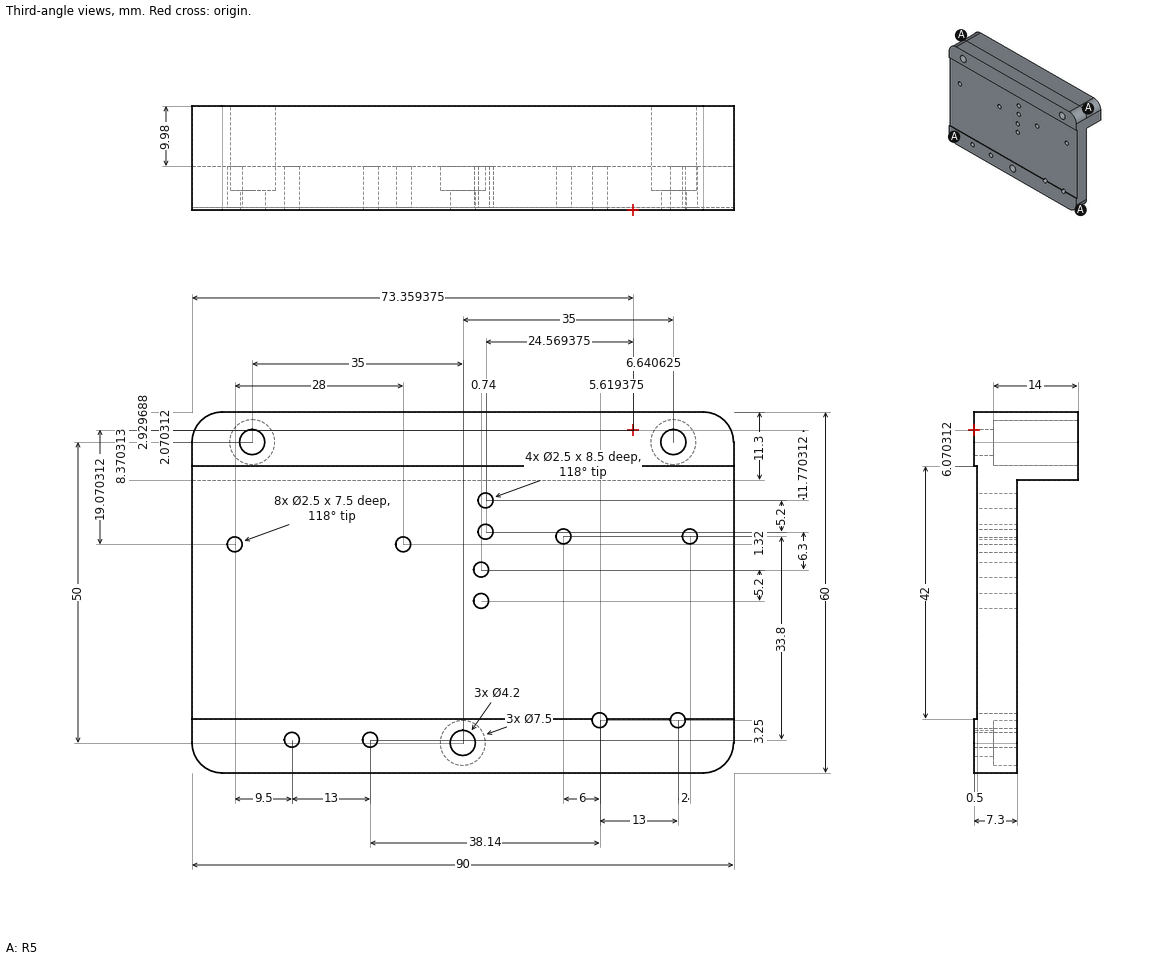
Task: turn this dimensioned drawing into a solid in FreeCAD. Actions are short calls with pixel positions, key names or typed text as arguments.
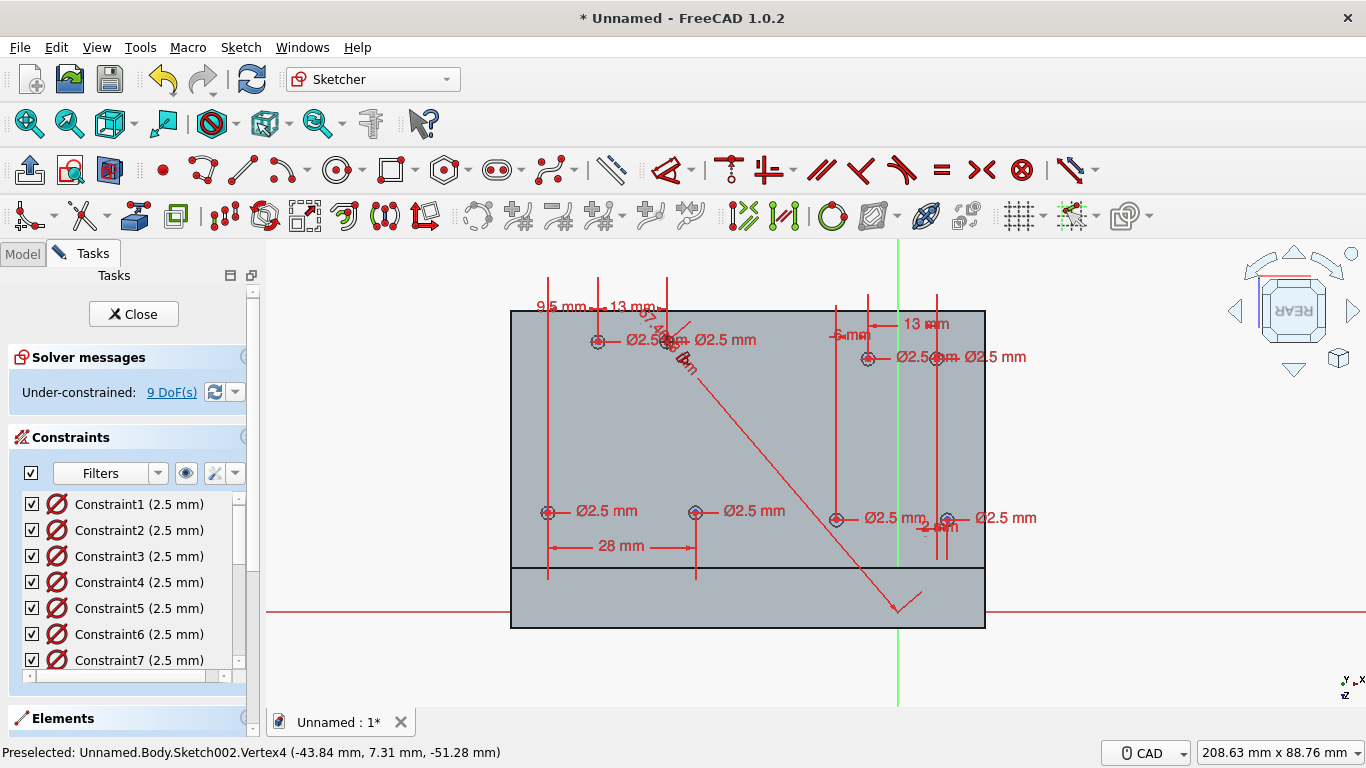
scroll(868, 359, up, 5)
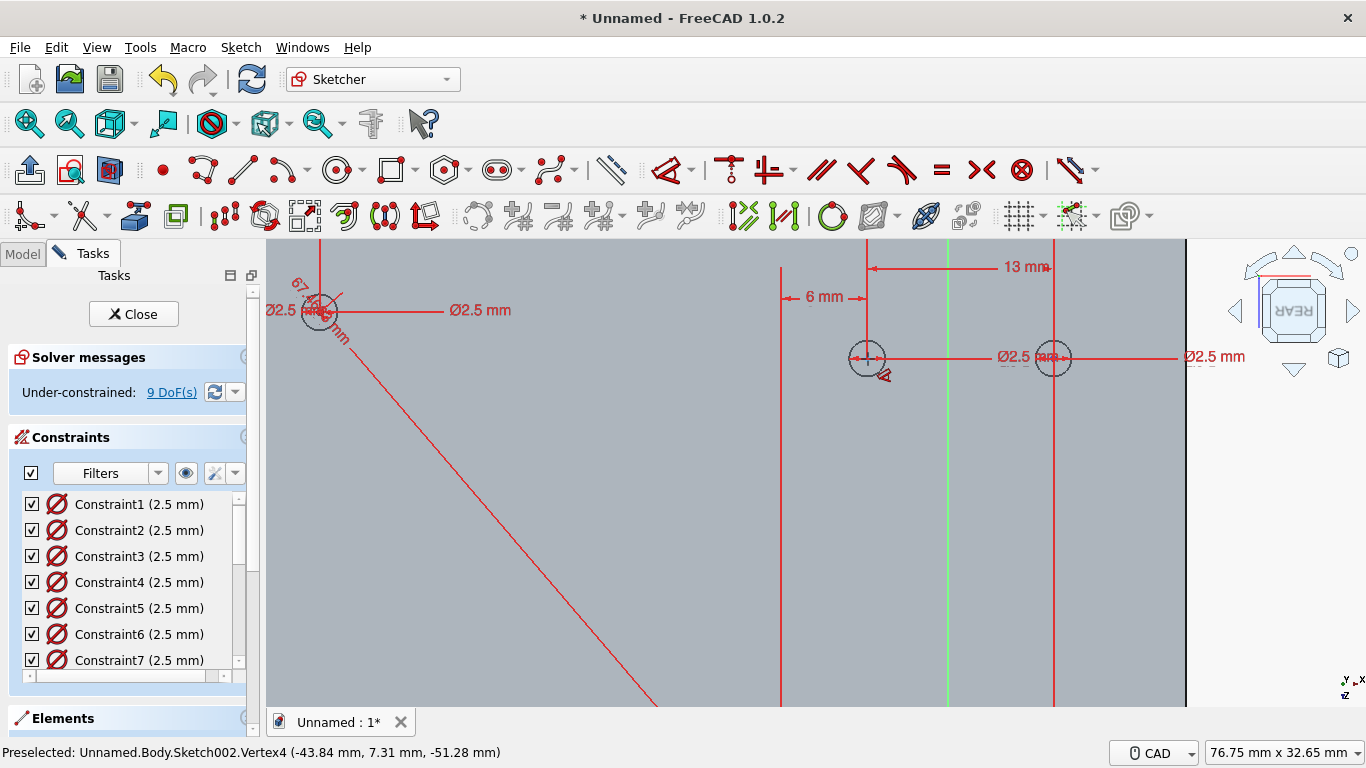
click(867, 359)
click(901, 335)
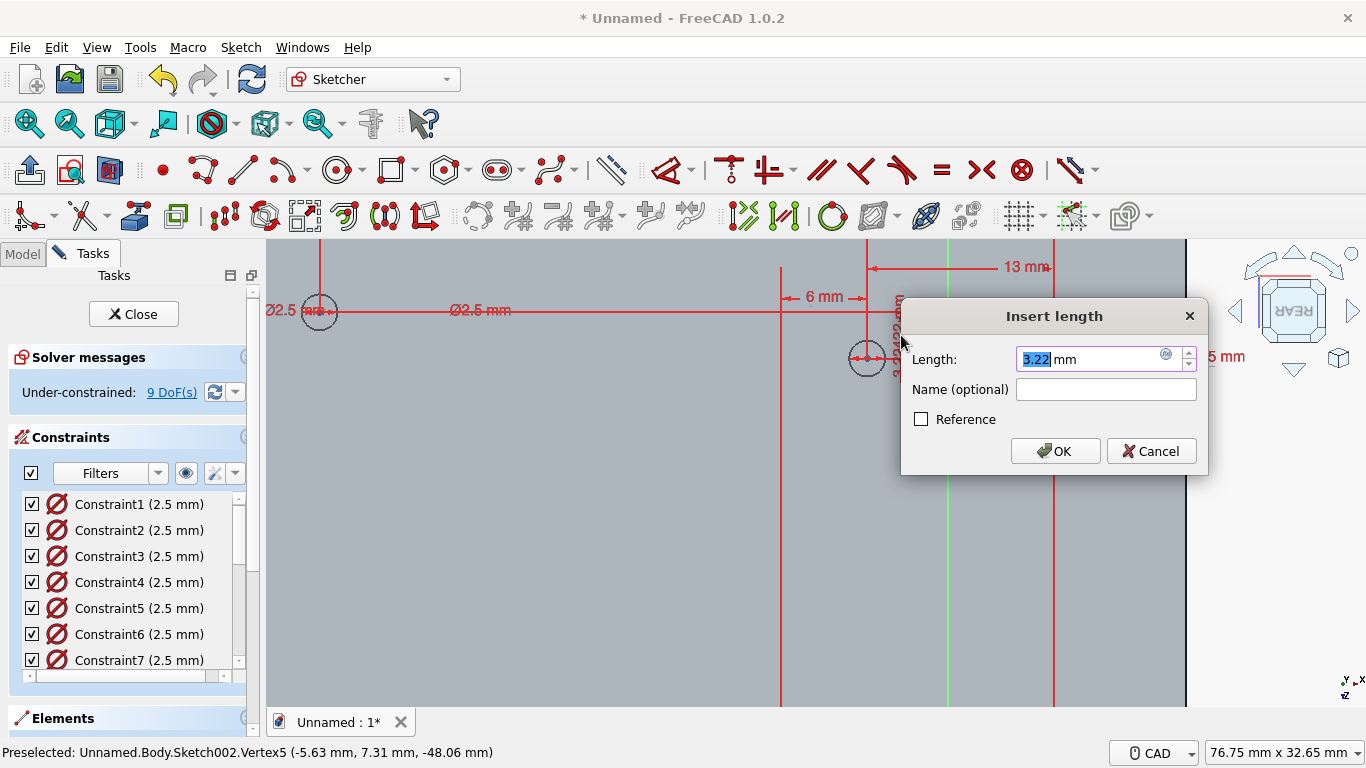
text(3.25)
key(Return)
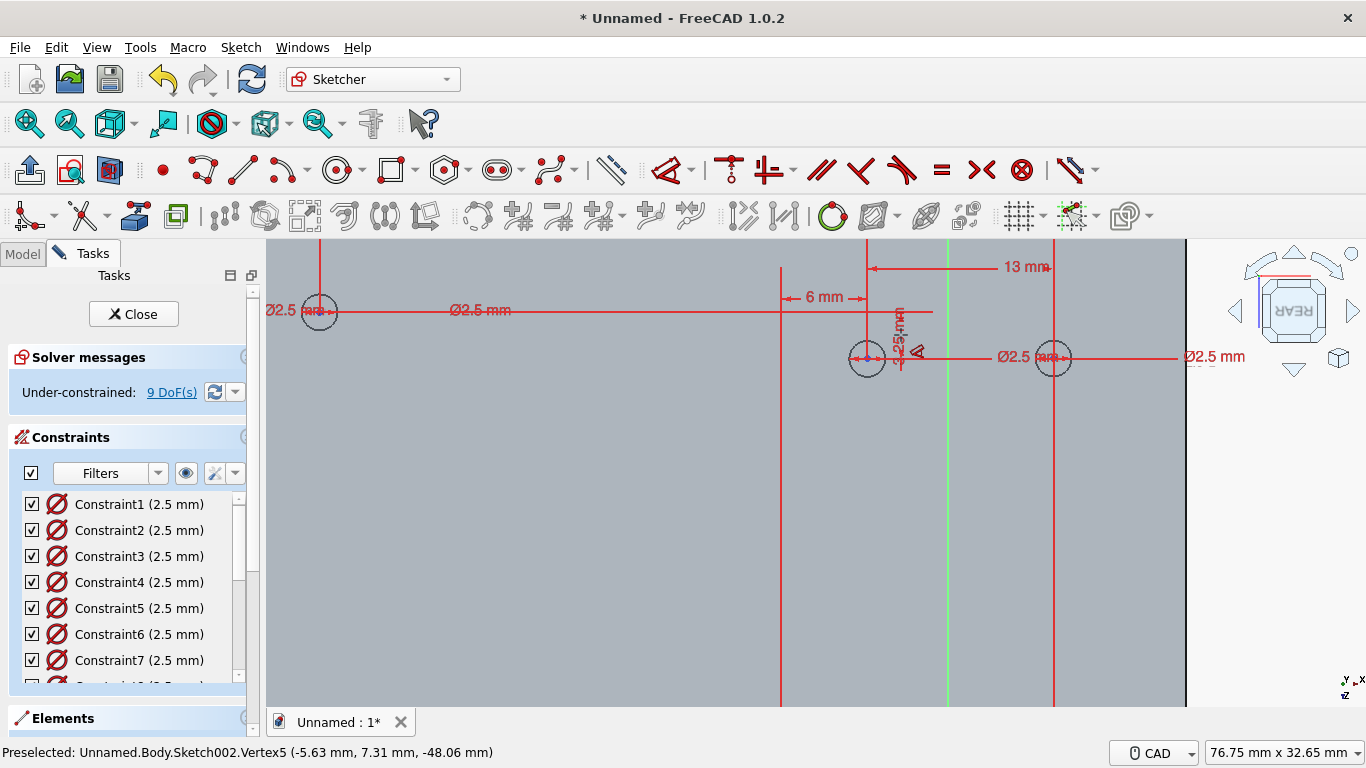
scroll(868, 359, down, 5)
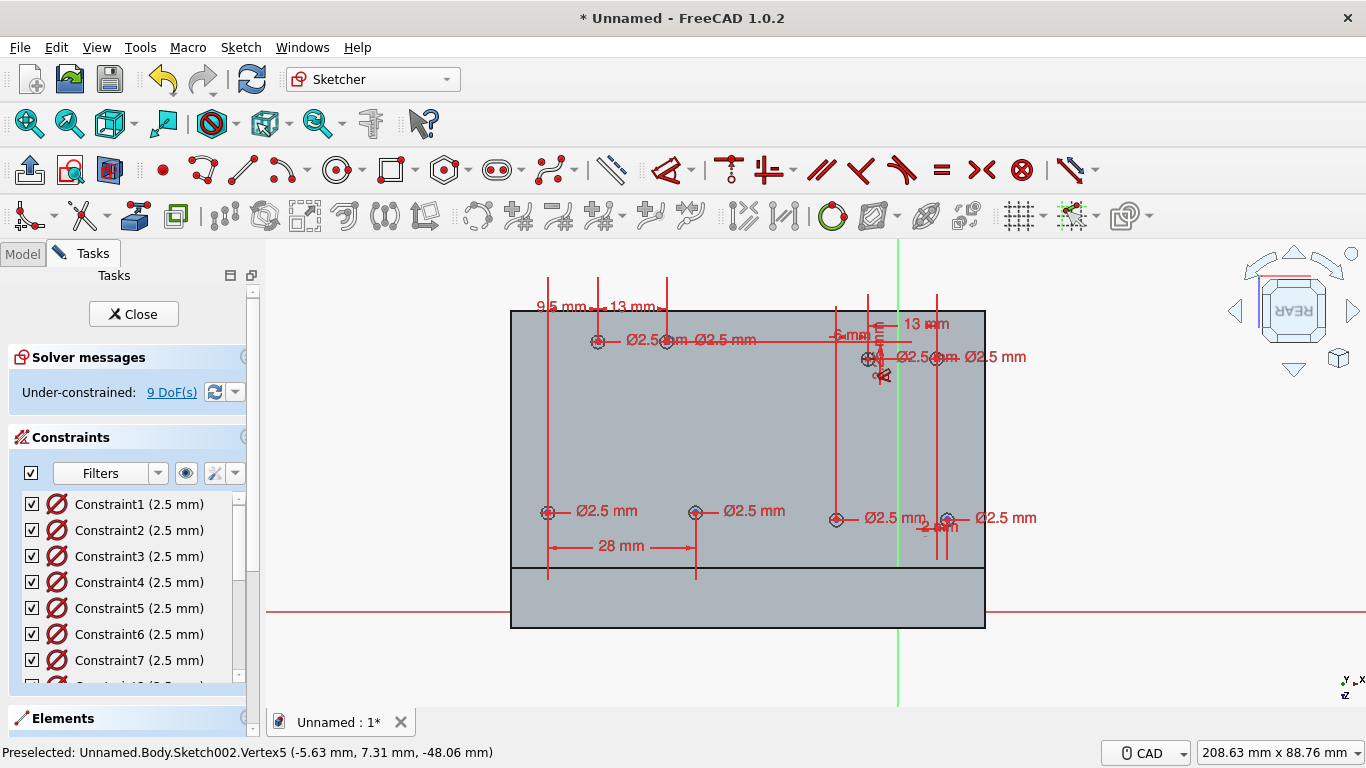
scroll(598, 342, up, 5)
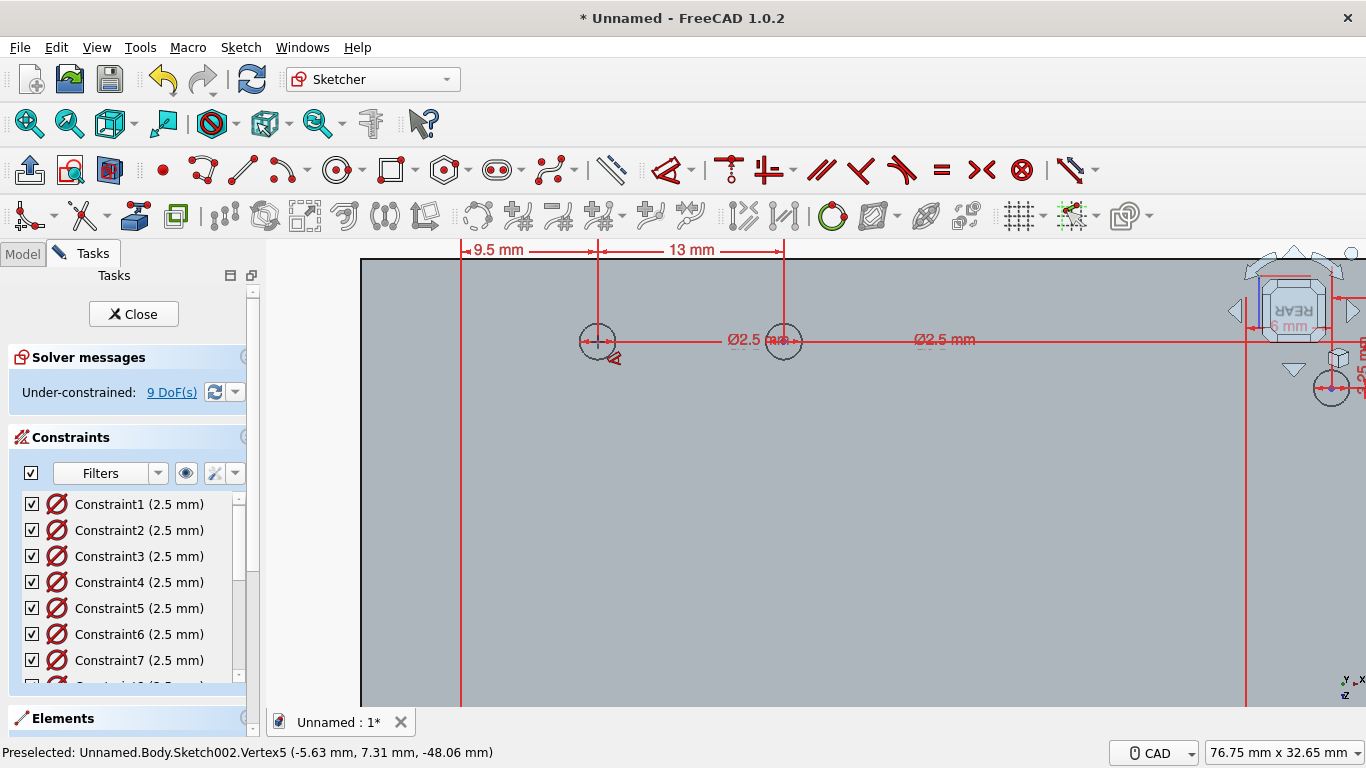
click(598, 342)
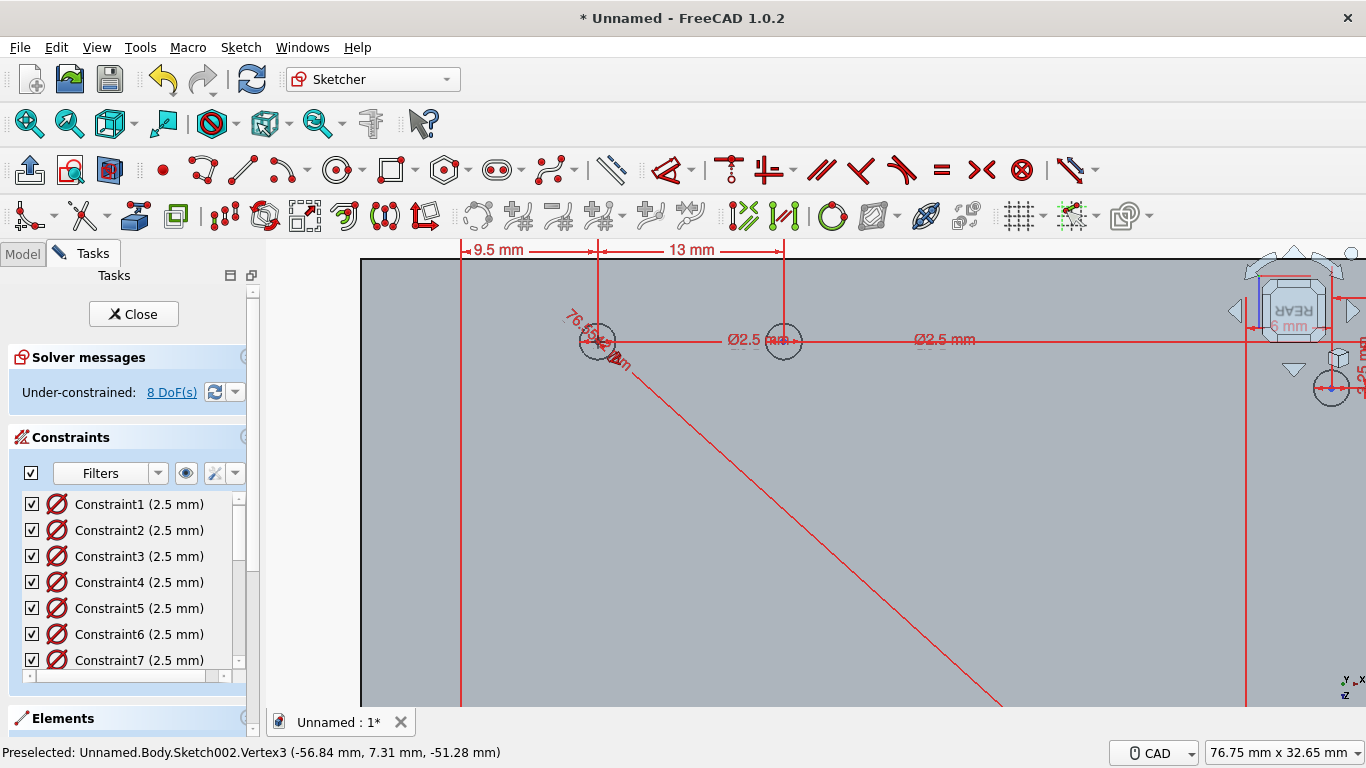
scroll(598, 342, down, 5)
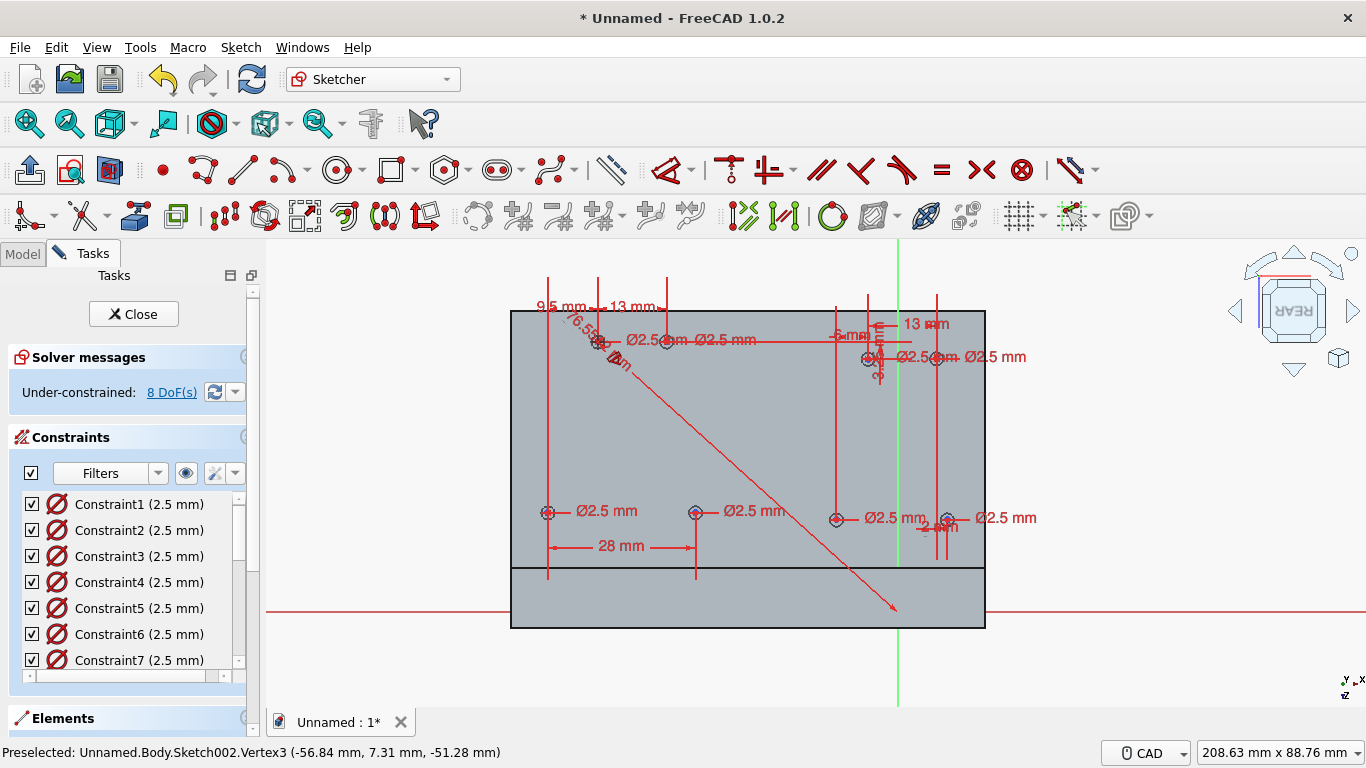
scroll(868, 359, up, 5)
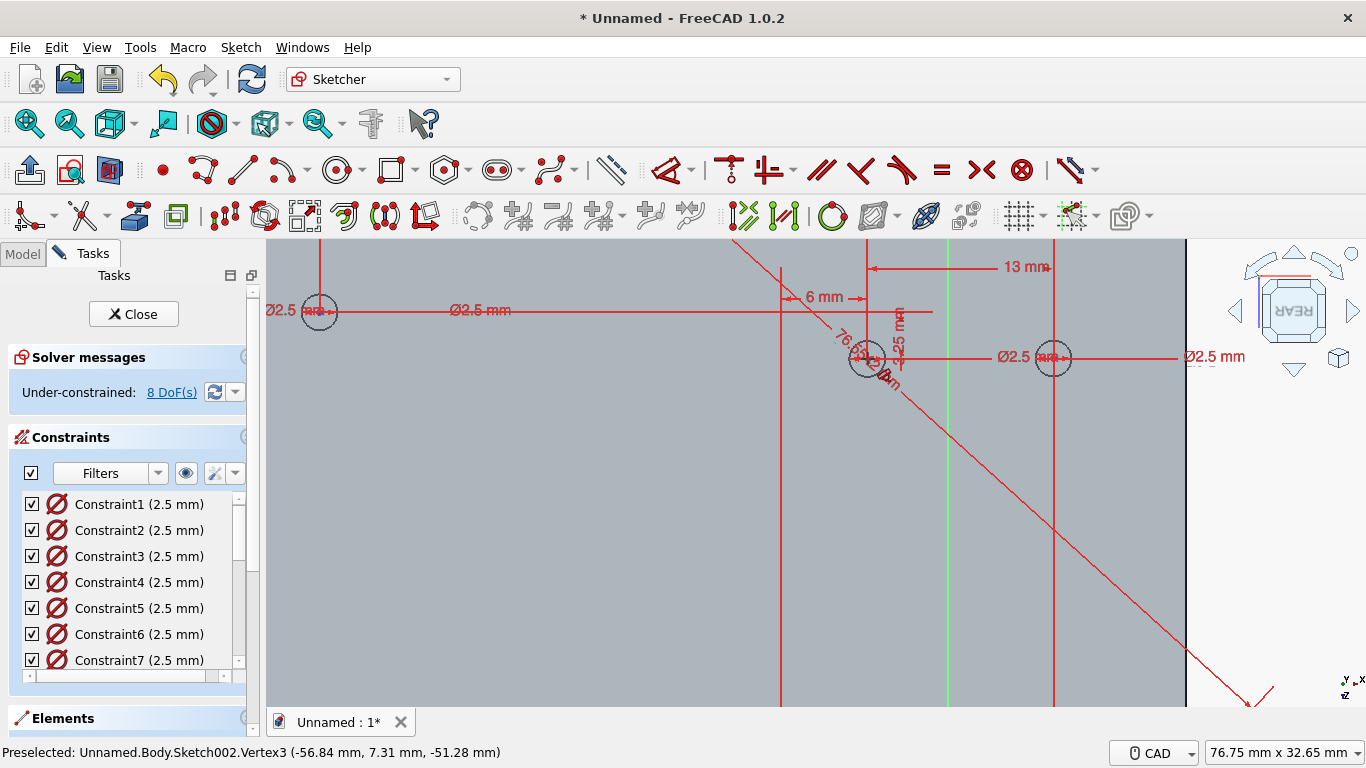
click(867, 359)
click(973, 336)